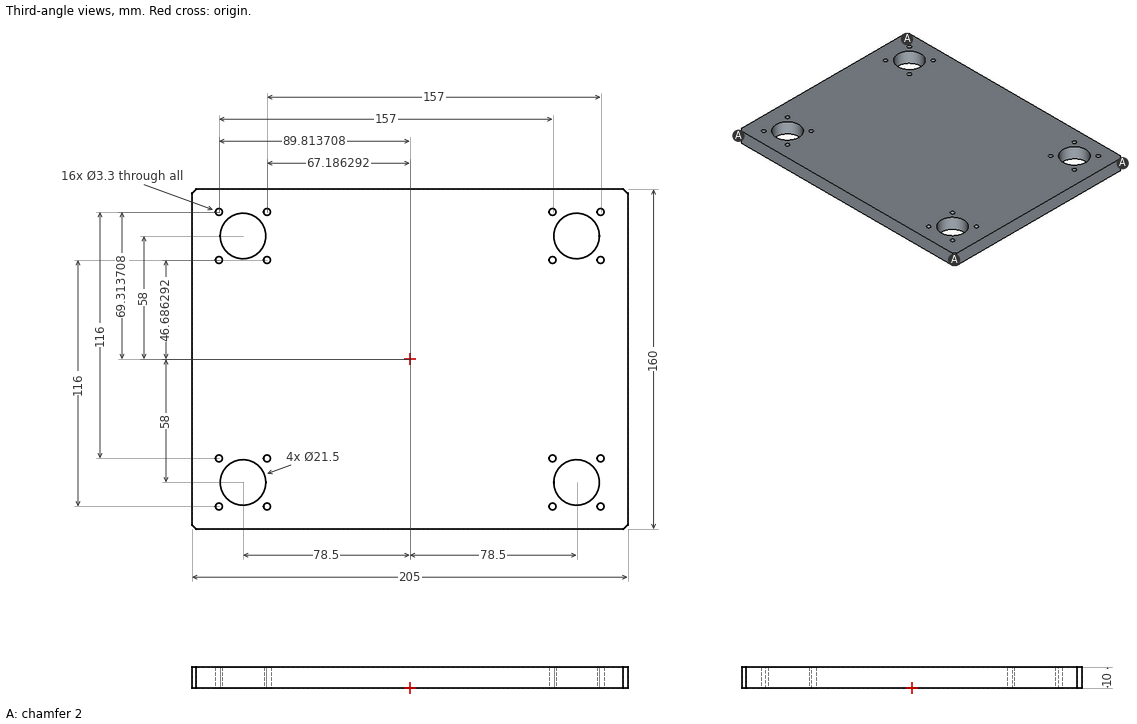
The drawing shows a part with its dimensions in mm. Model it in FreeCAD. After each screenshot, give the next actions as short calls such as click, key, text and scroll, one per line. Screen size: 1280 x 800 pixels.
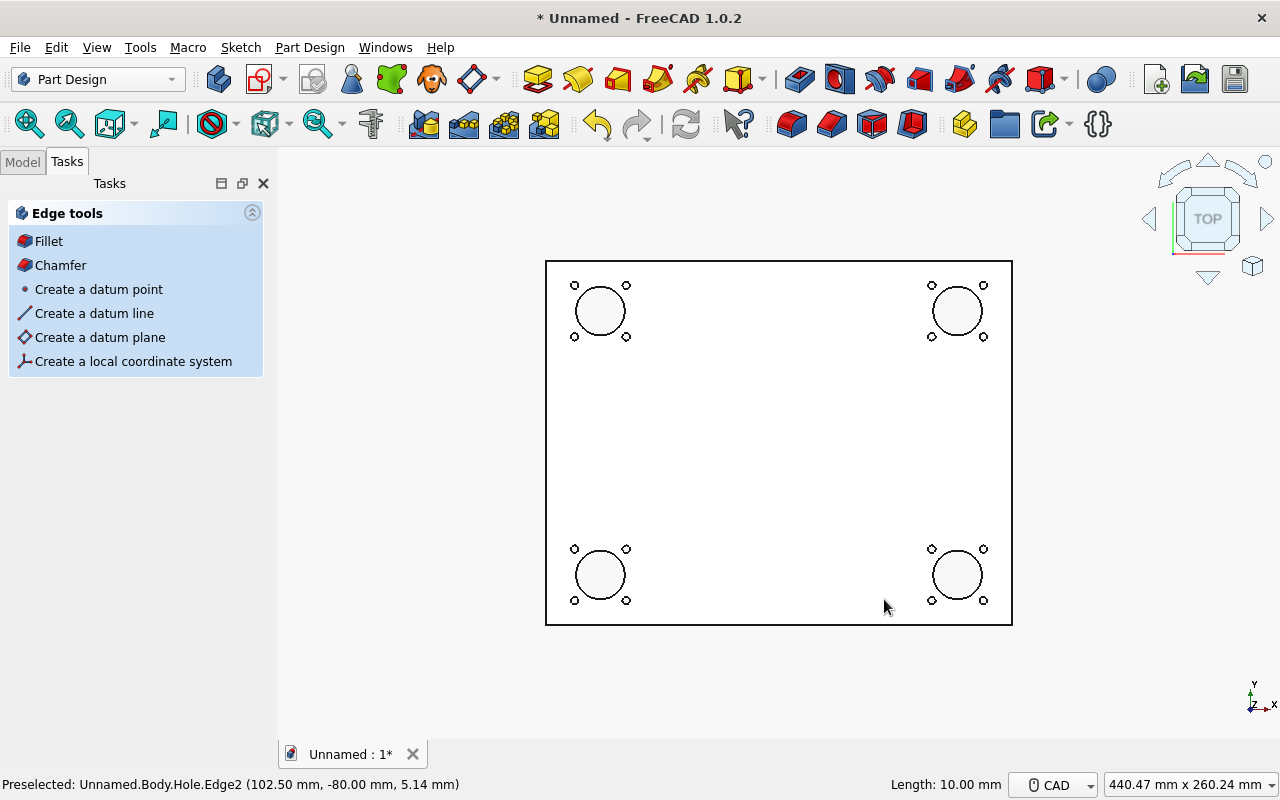
key(1)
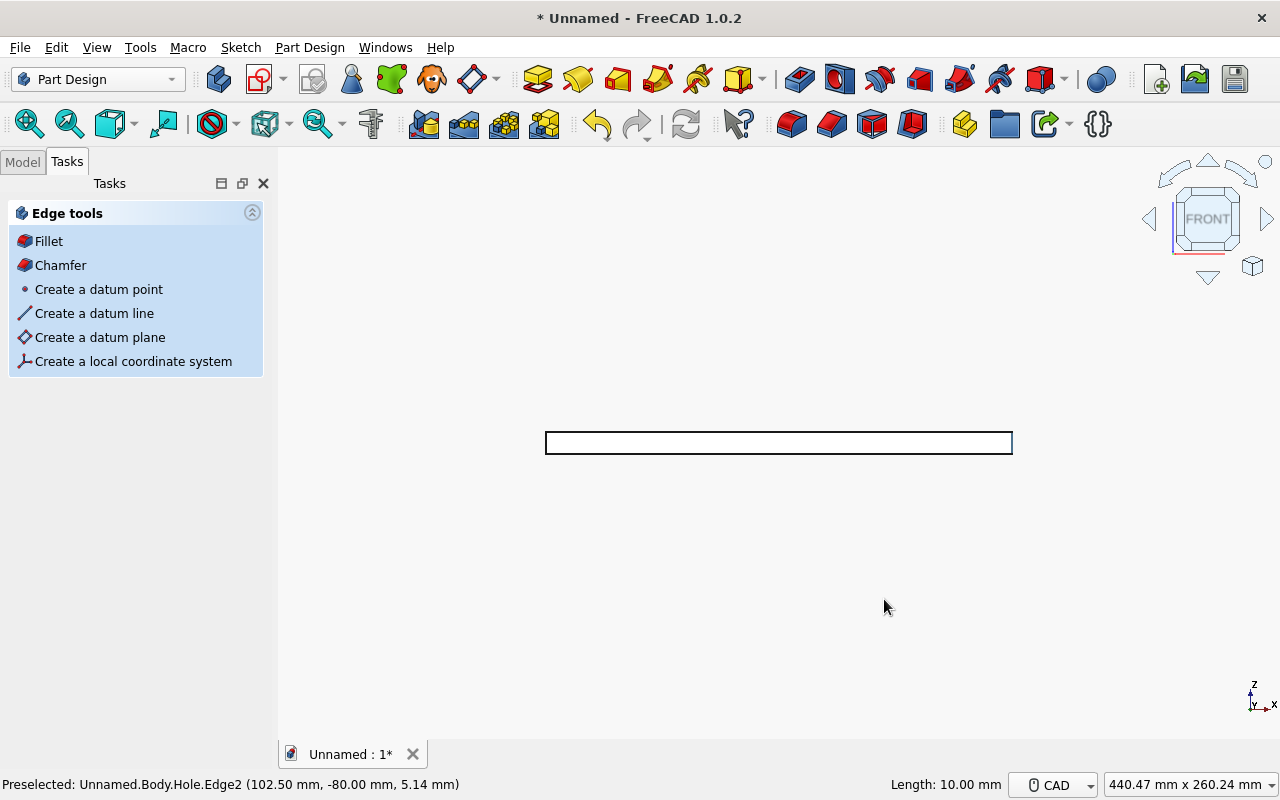
click(546, 442, ctrl)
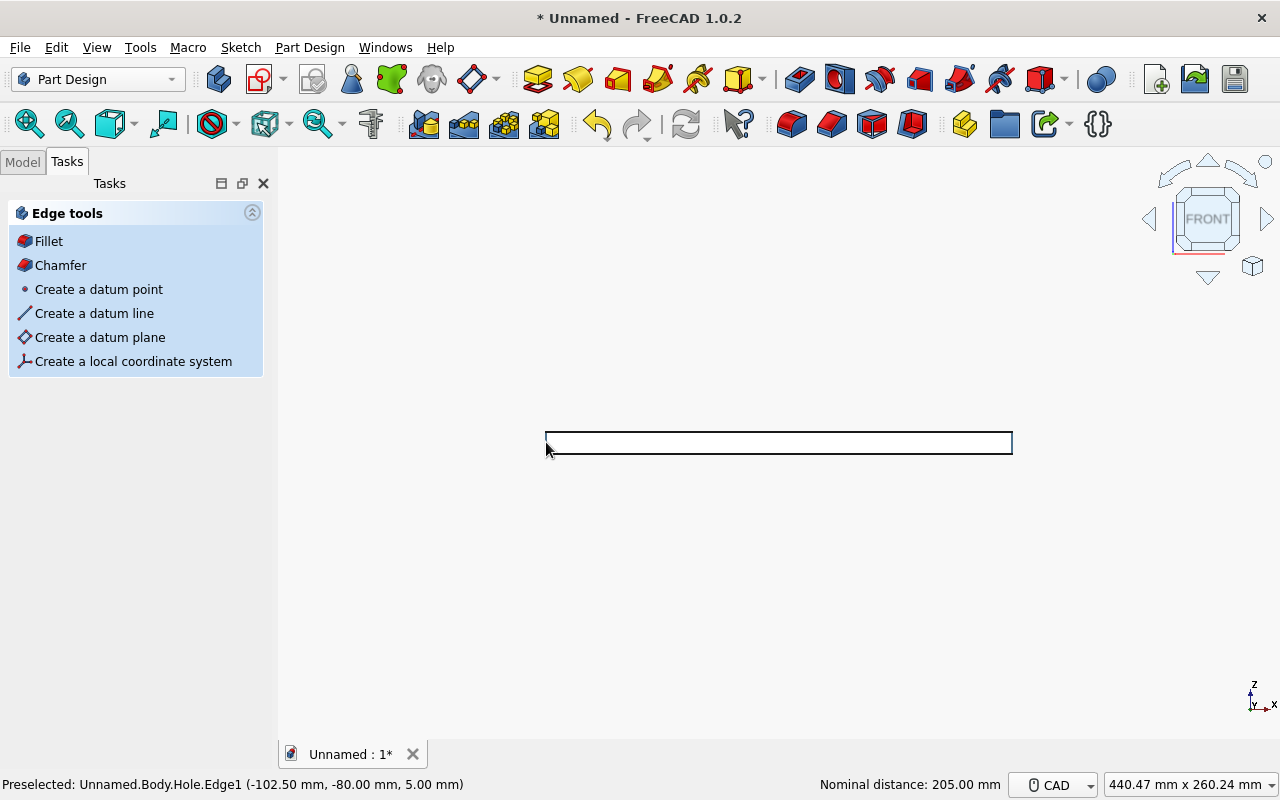
key(3)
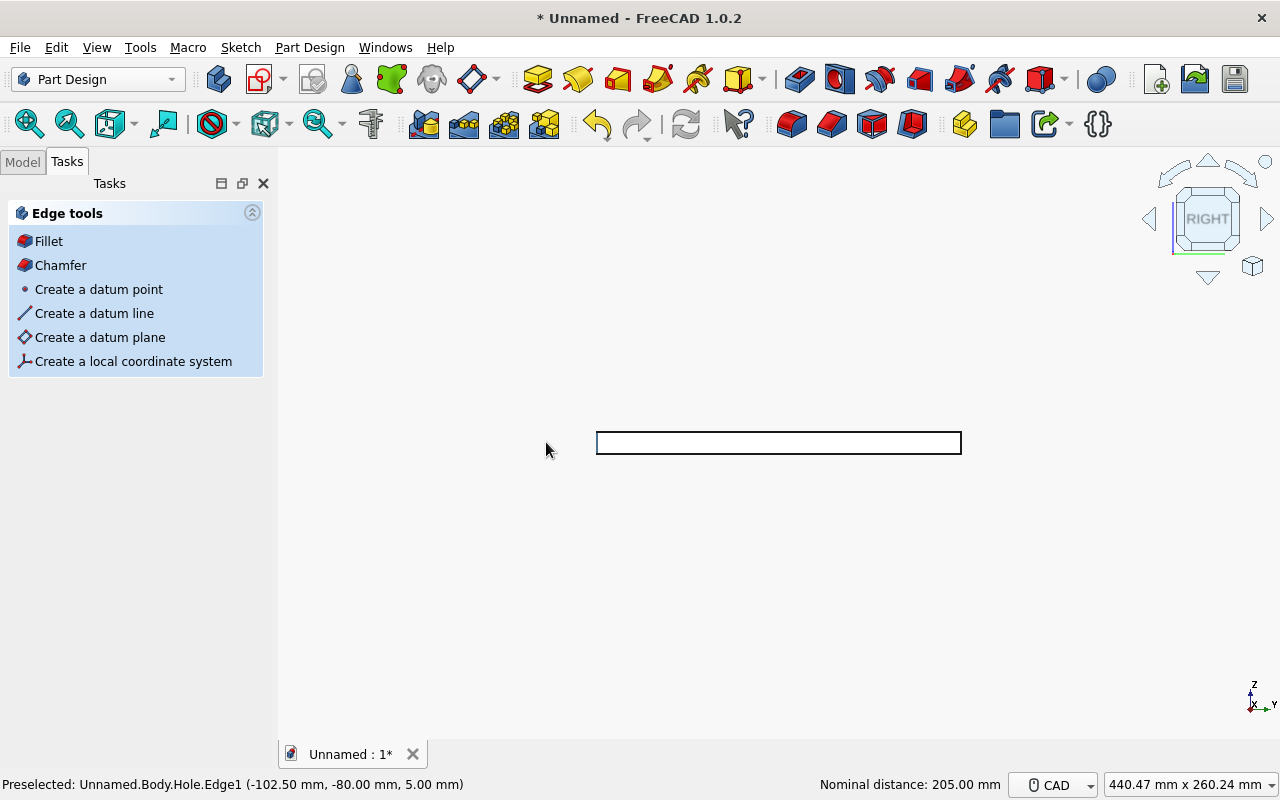
click(30, 124)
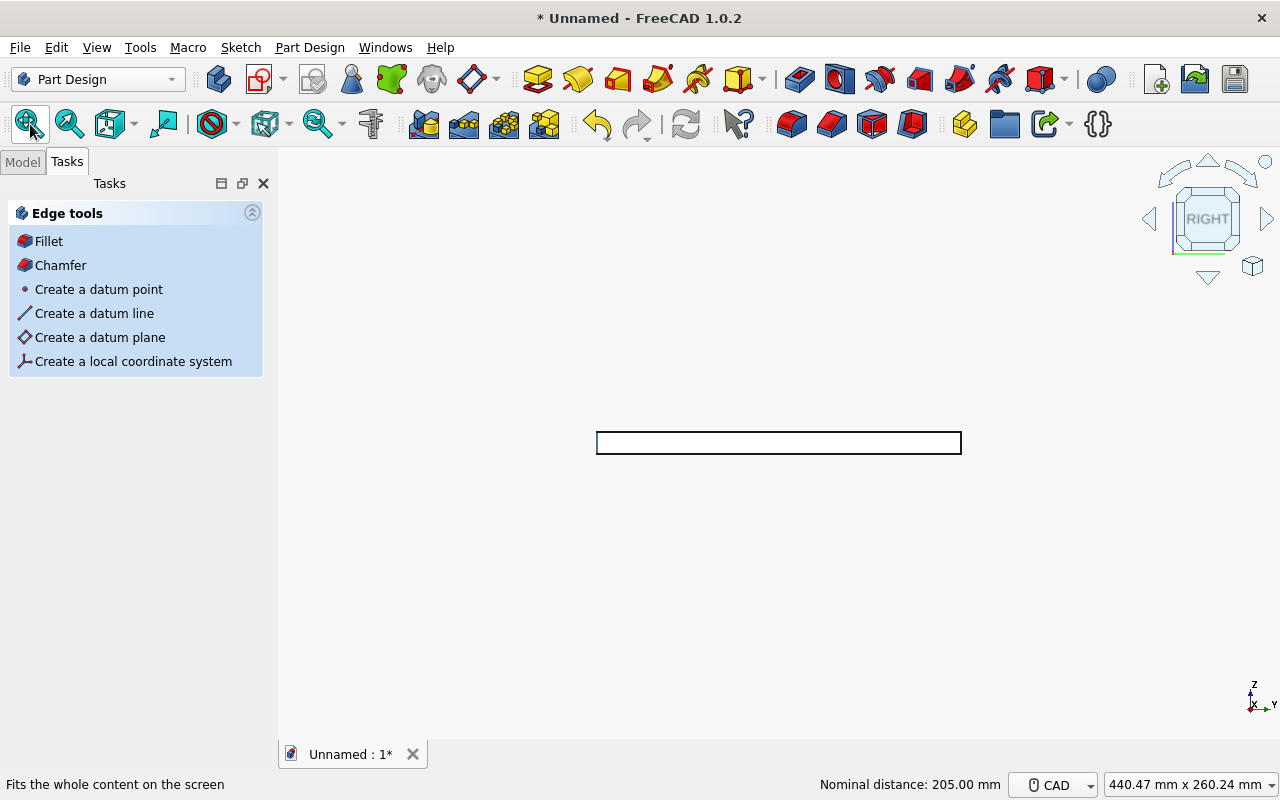
click(961, 442, ctrl)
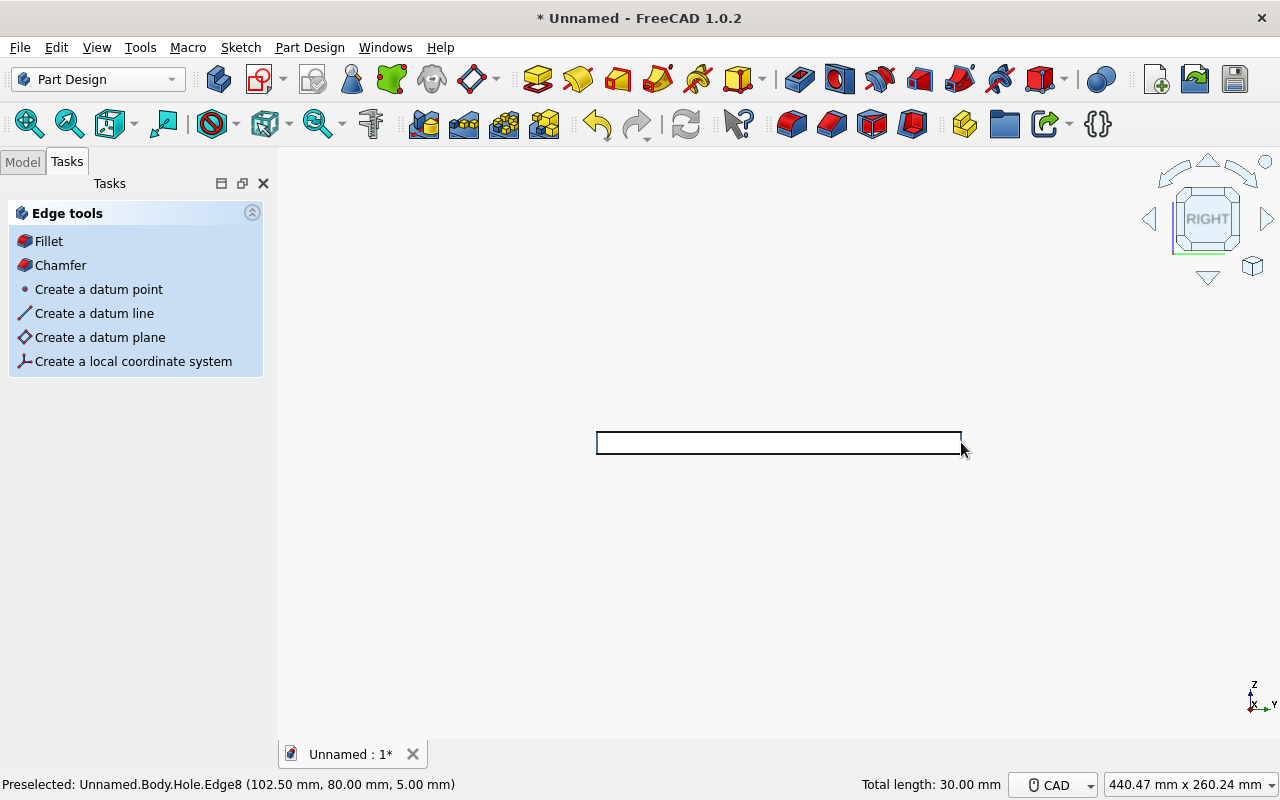
key(5)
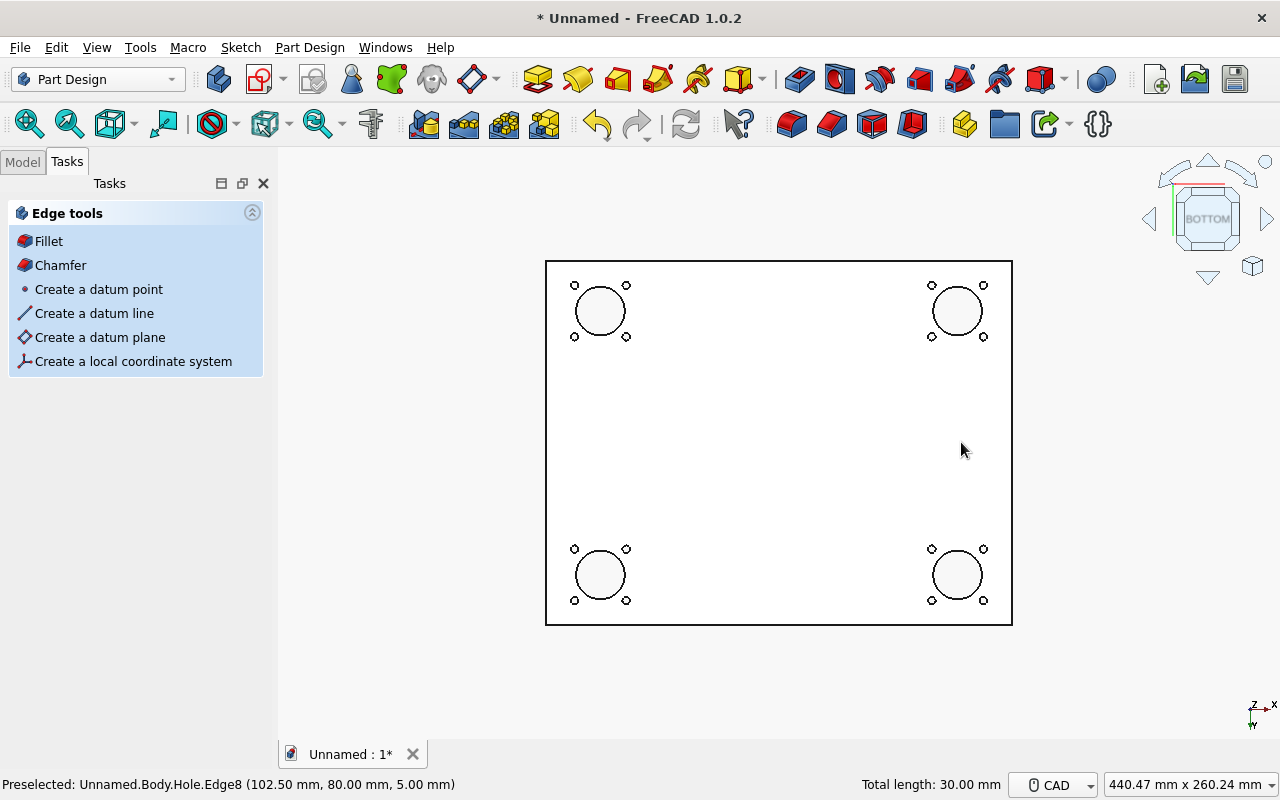
key(4)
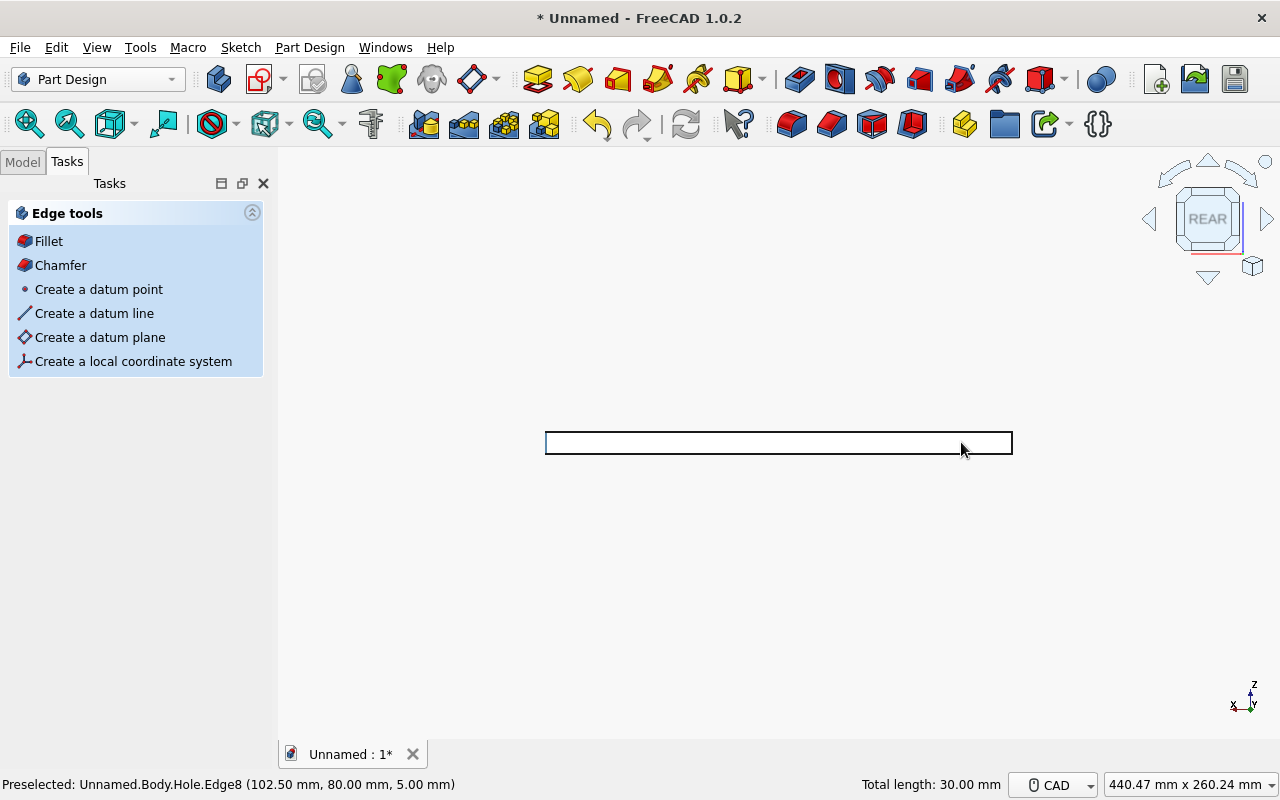
click(1012, 442, ctrl)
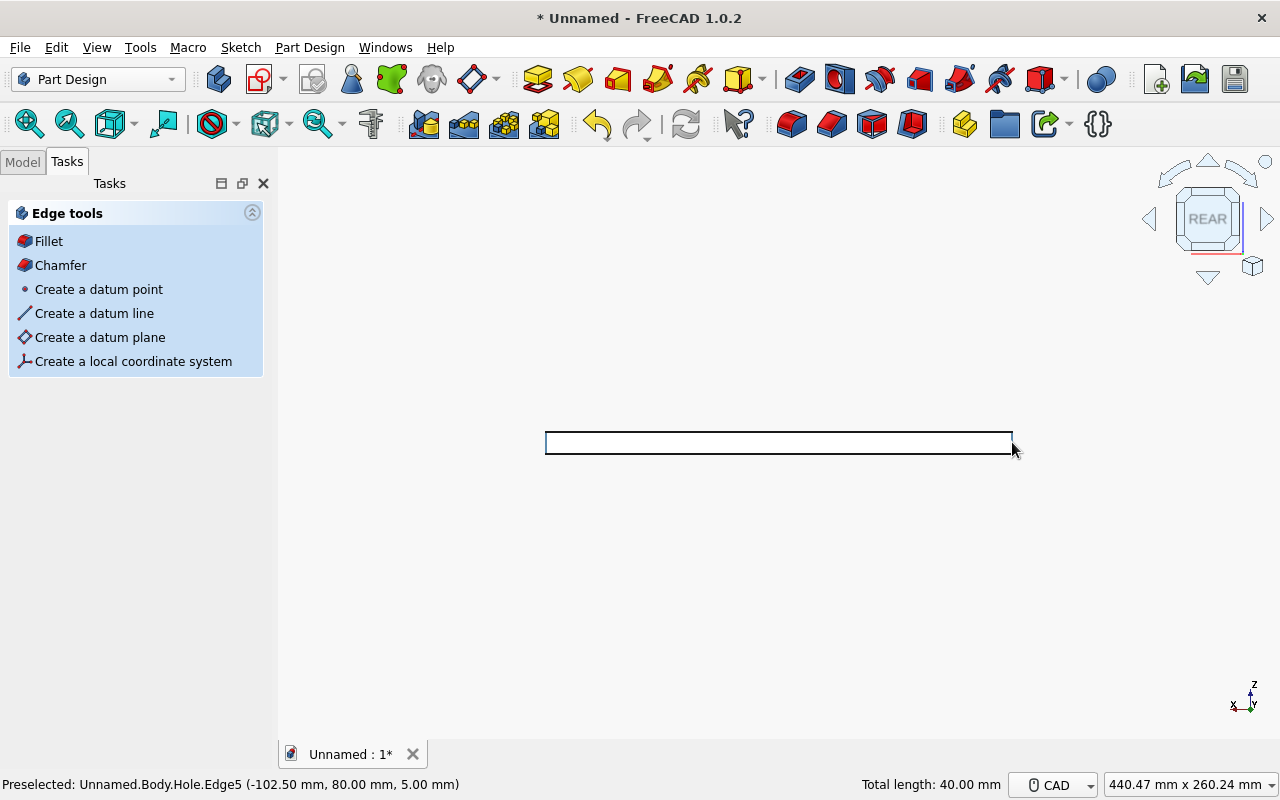
click(832, 124)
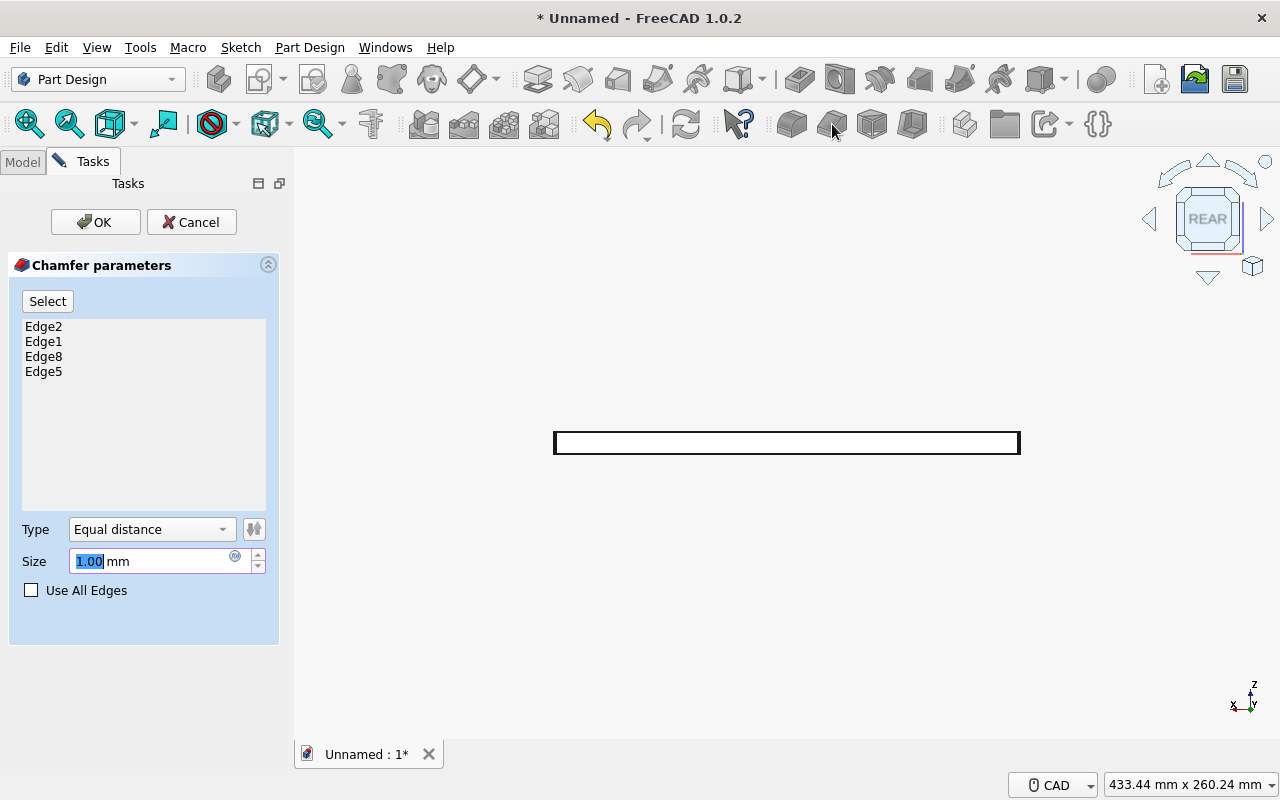
text(2)
key(Tab)